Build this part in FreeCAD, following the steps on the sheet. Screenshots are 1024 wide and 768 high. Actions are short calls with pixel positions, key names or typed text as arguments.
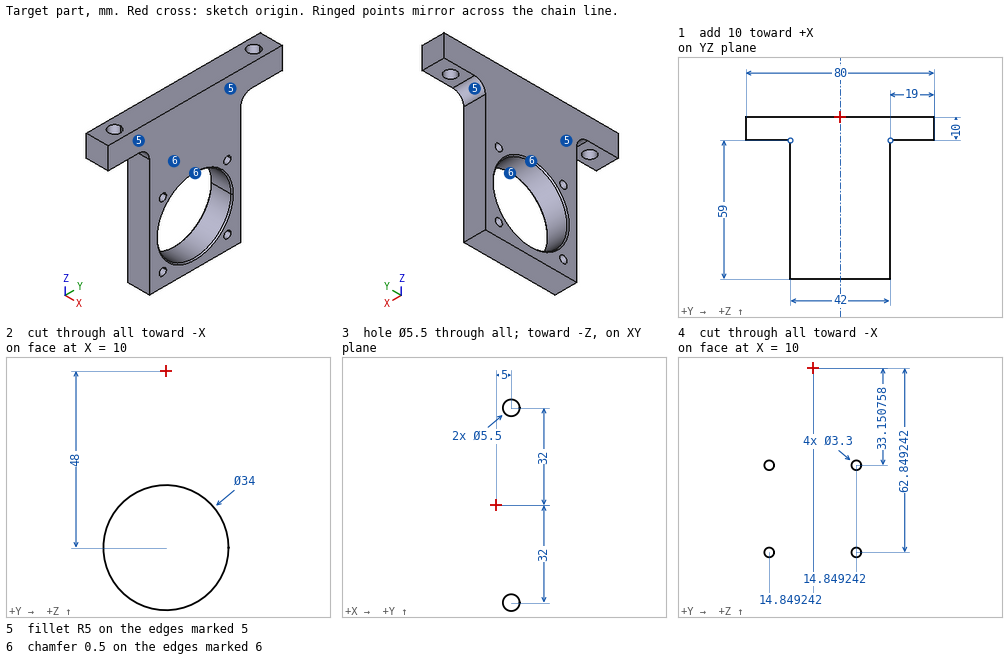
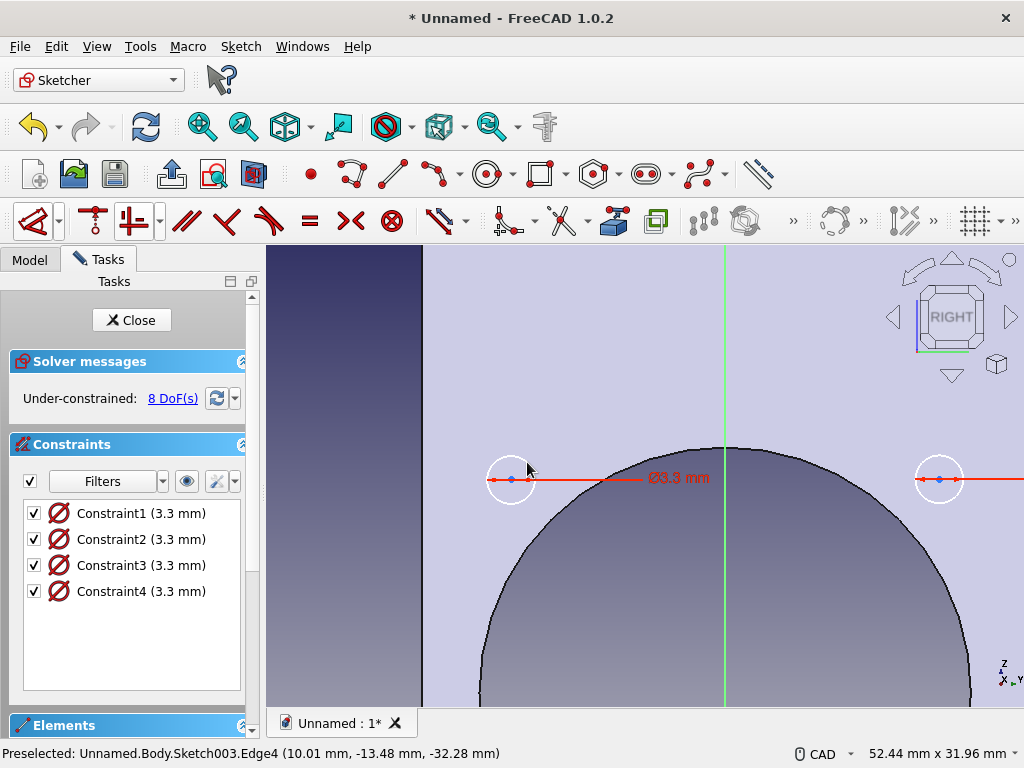
scroll(512, 480, down, 6)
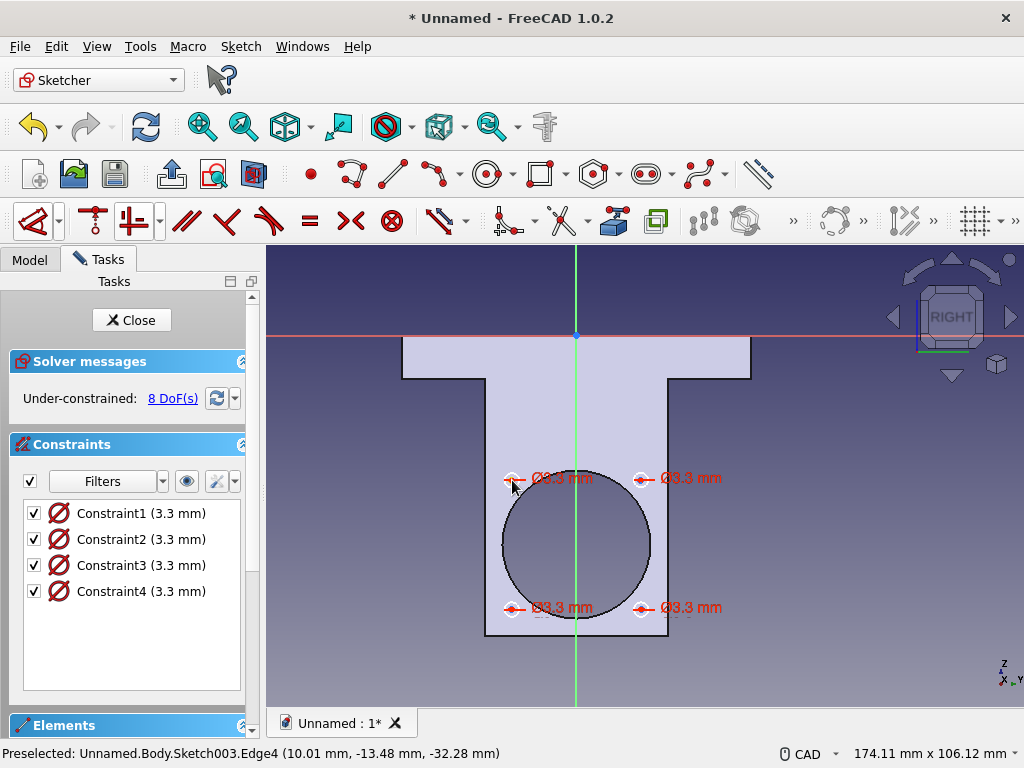
click(641, 480)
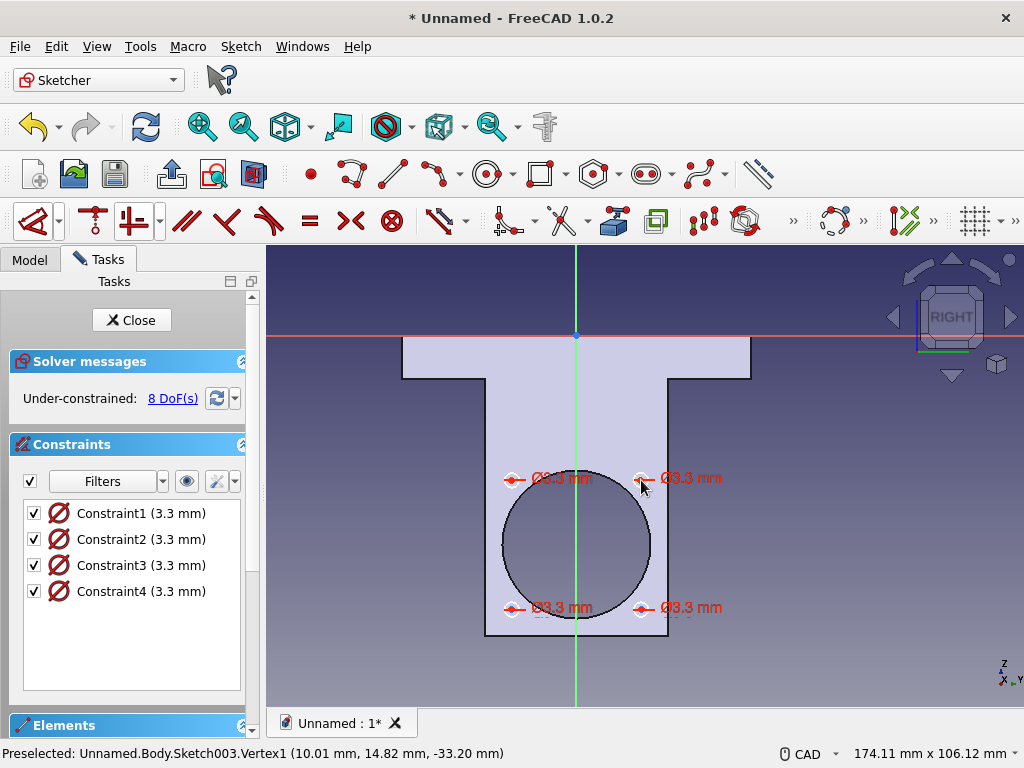
click(641, 610)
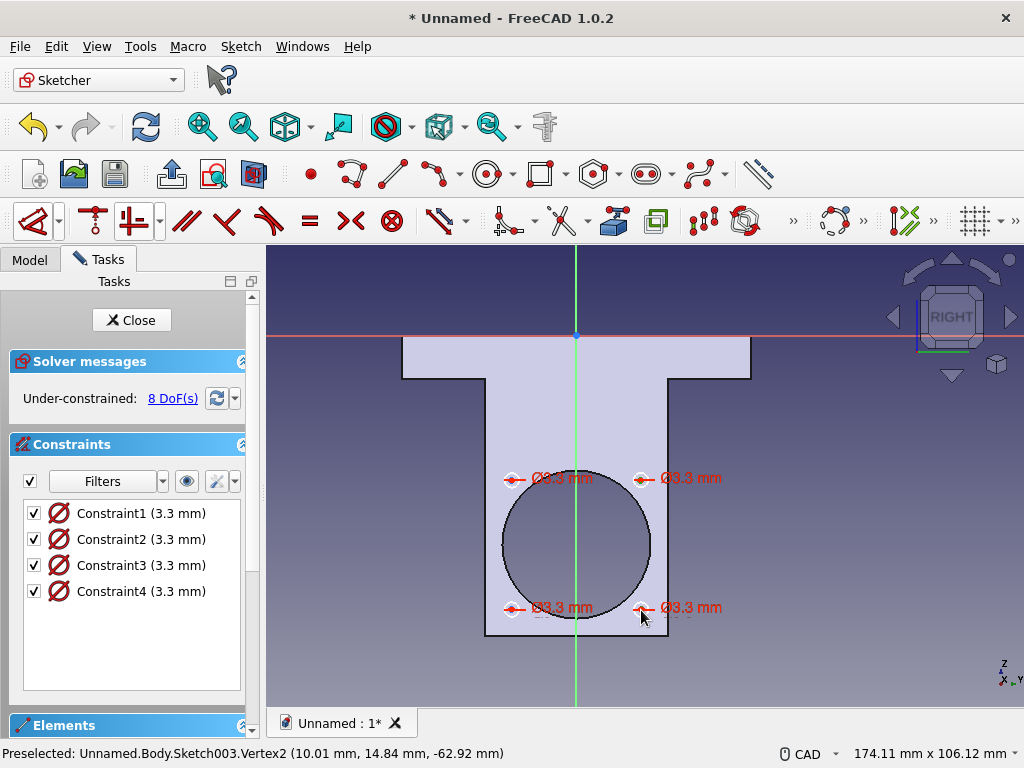
click(160, 222)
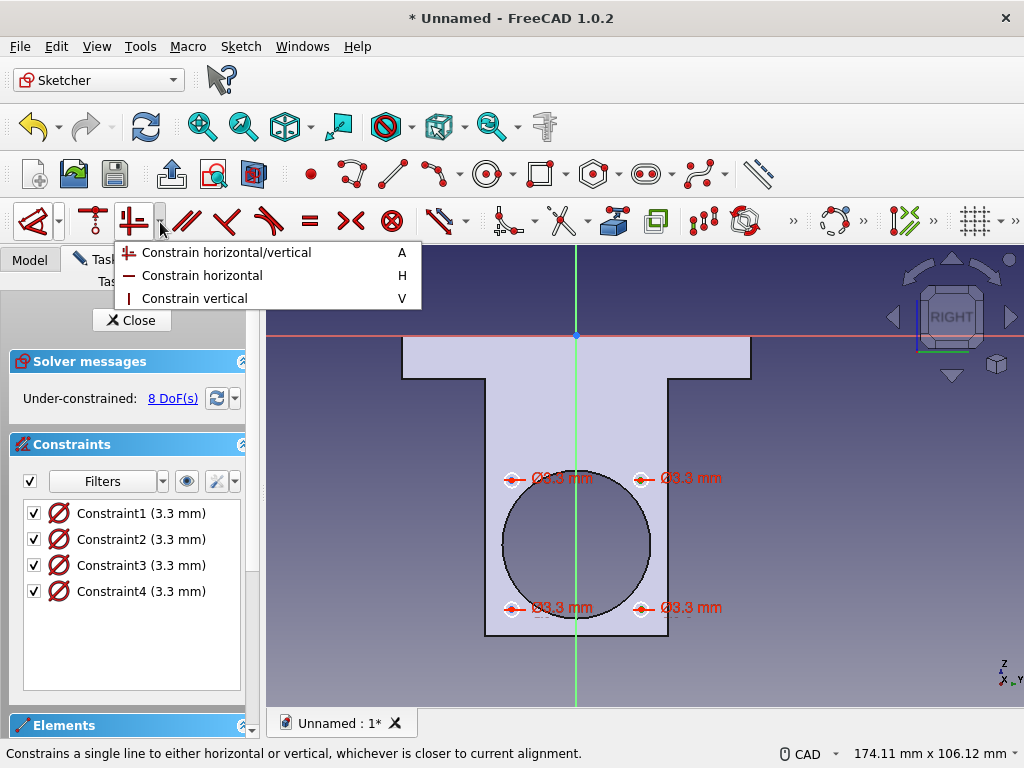
click(268, 298)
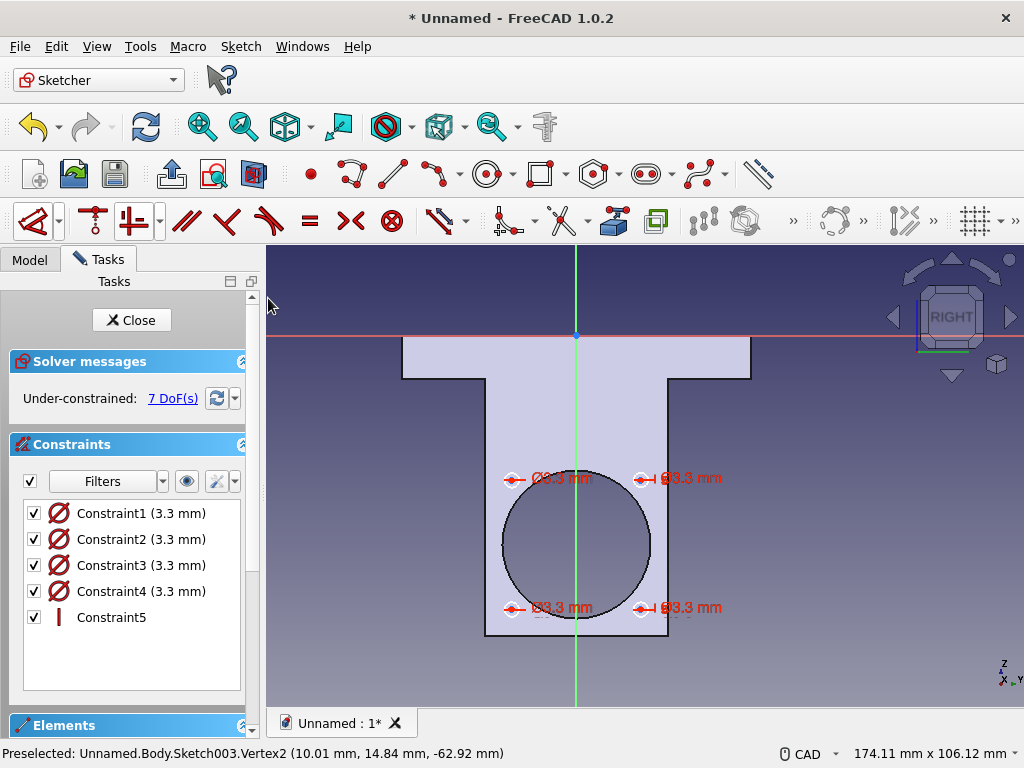
click(641, 610)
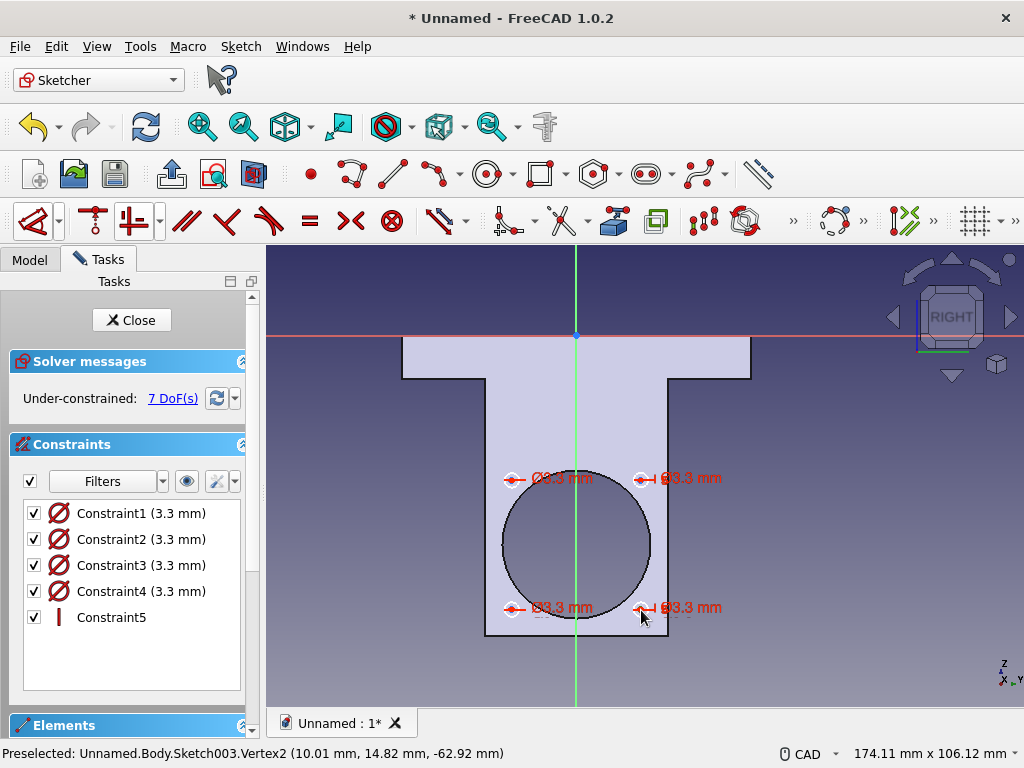
click(512, 610)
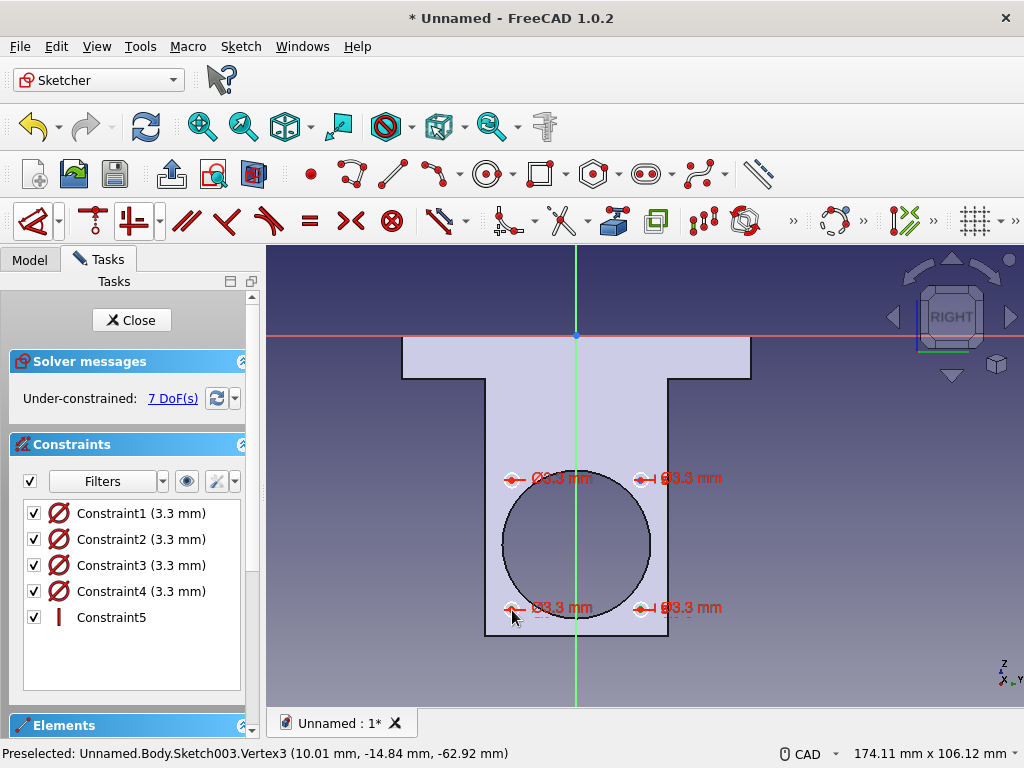
click(160, 222)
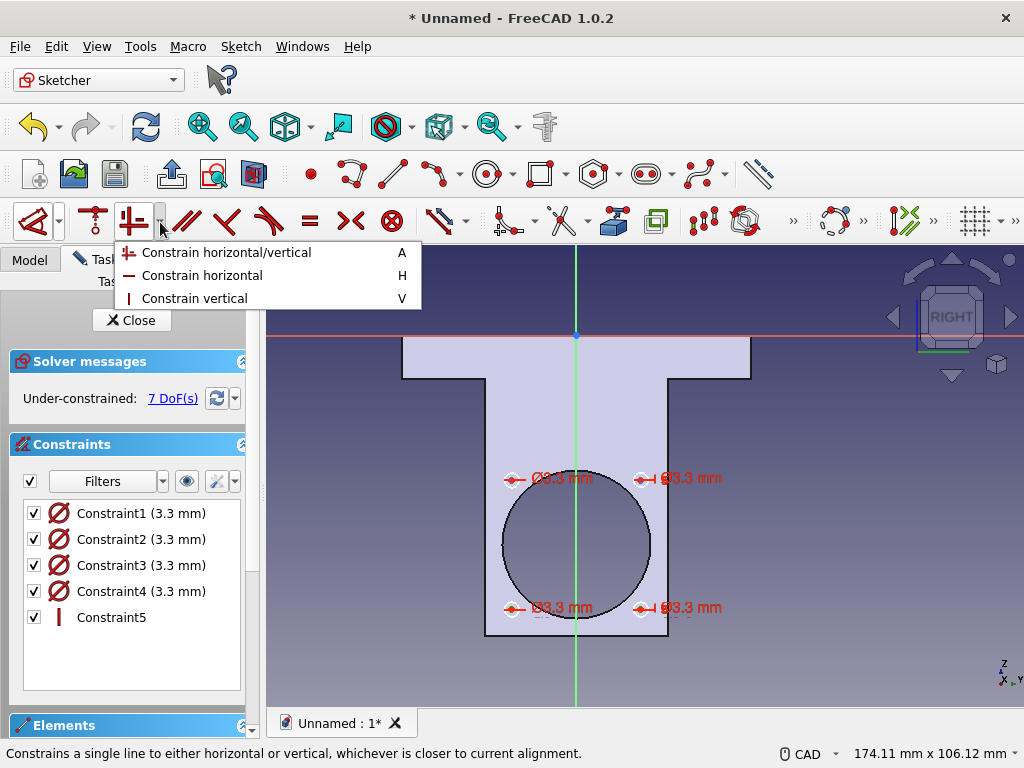
click(268, 276)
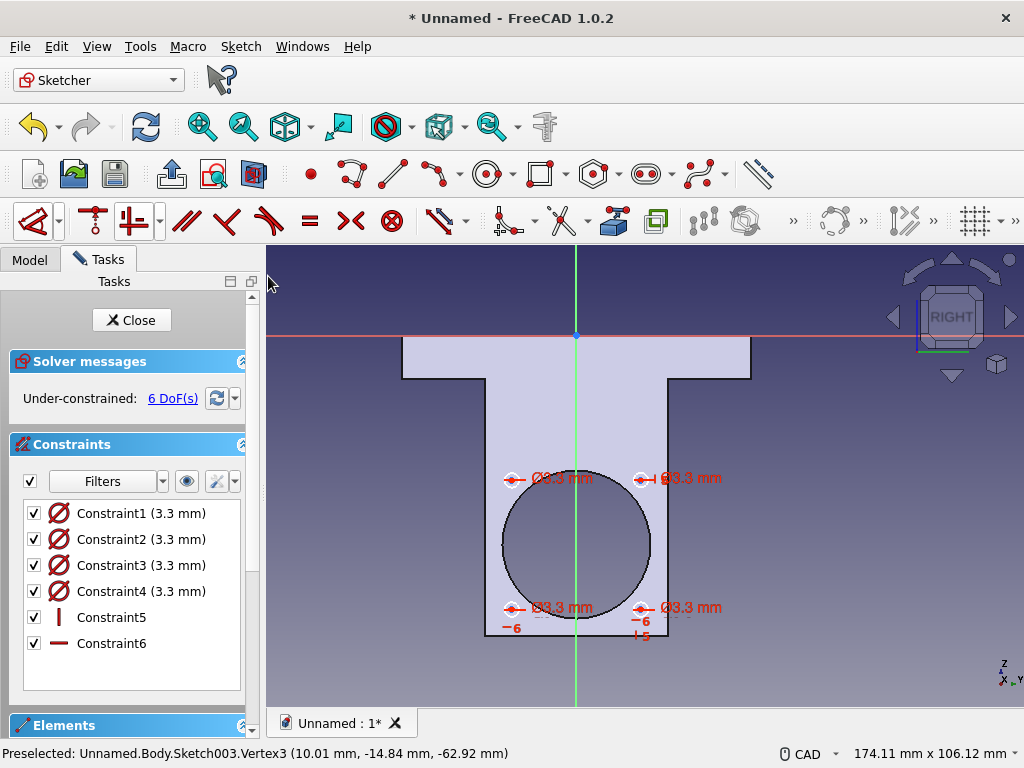
click(512, 610)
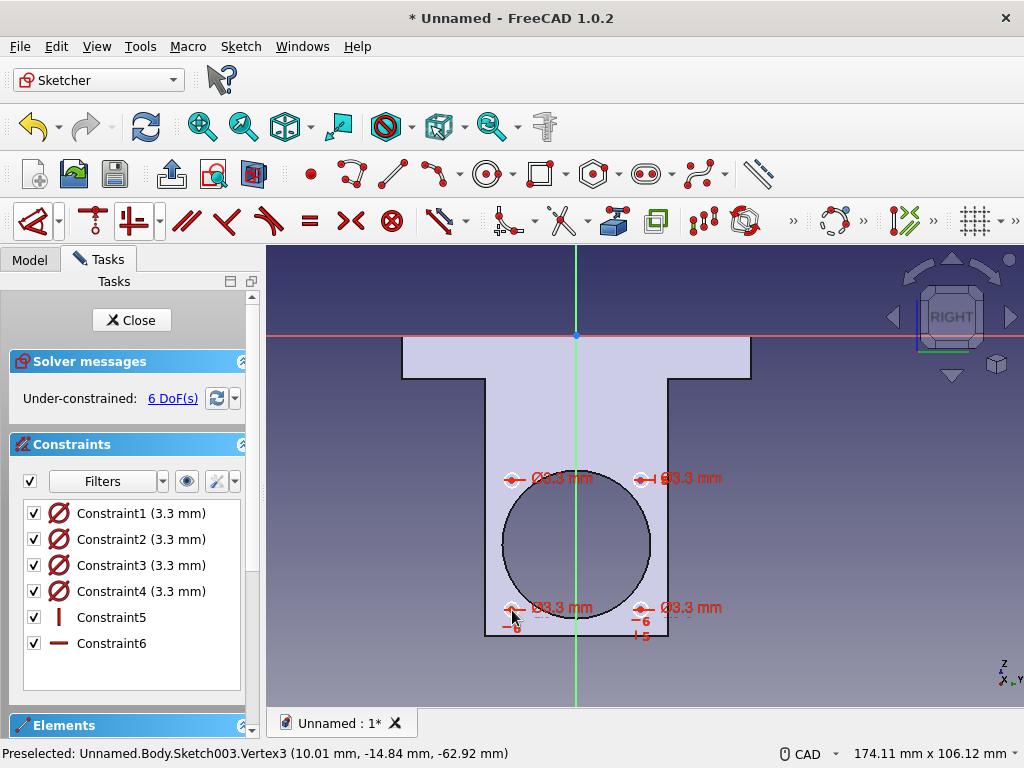
click(512, 480)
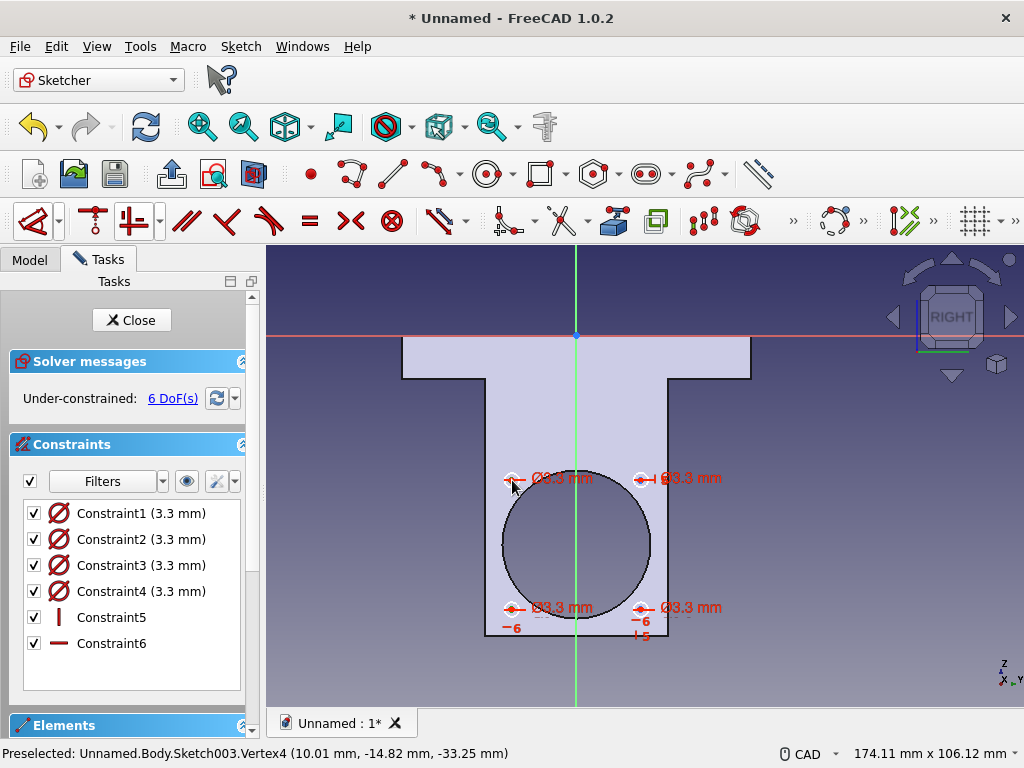
click(160, 222)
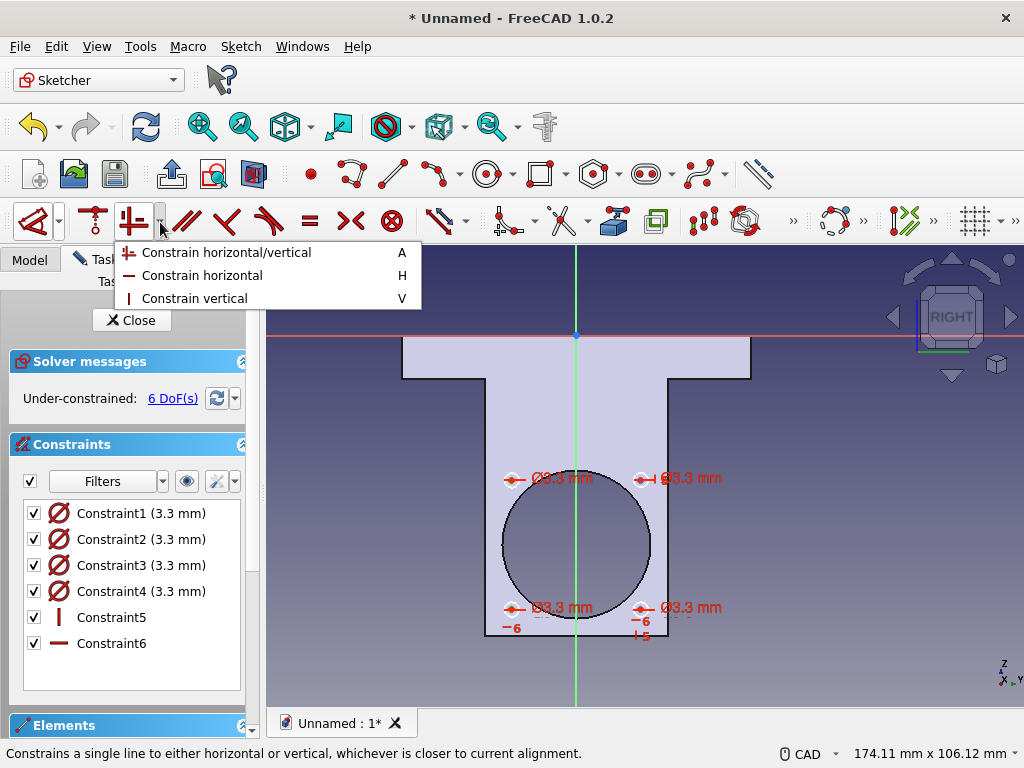
click(268, 298)